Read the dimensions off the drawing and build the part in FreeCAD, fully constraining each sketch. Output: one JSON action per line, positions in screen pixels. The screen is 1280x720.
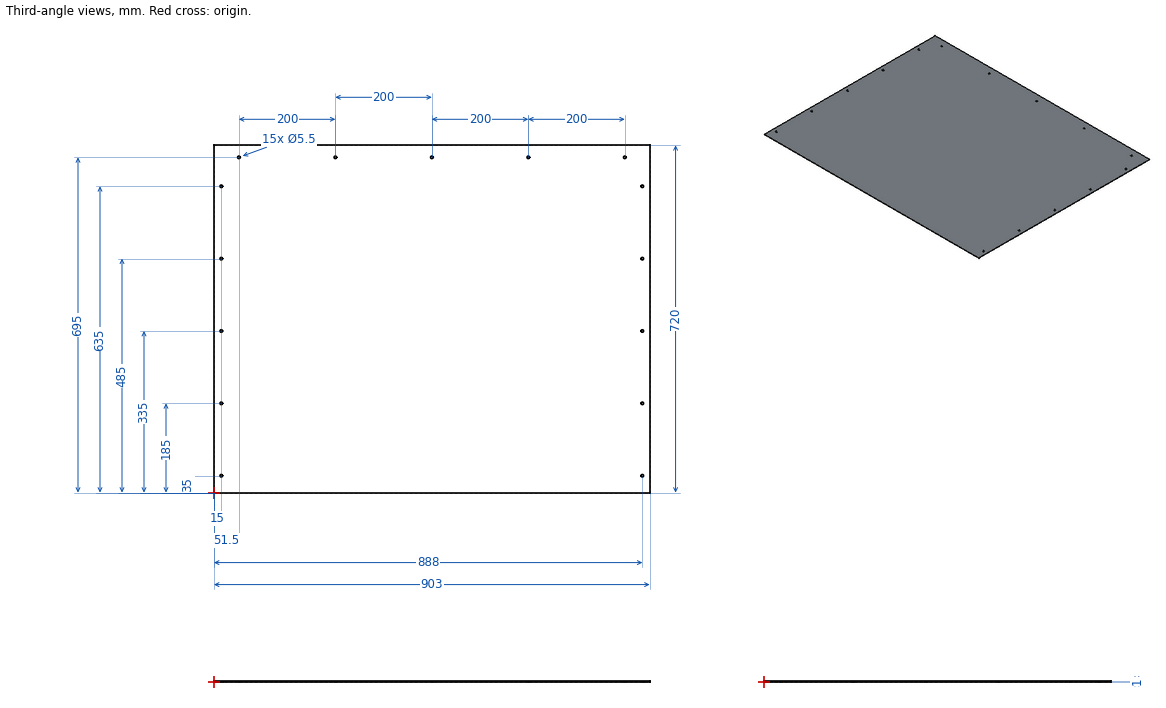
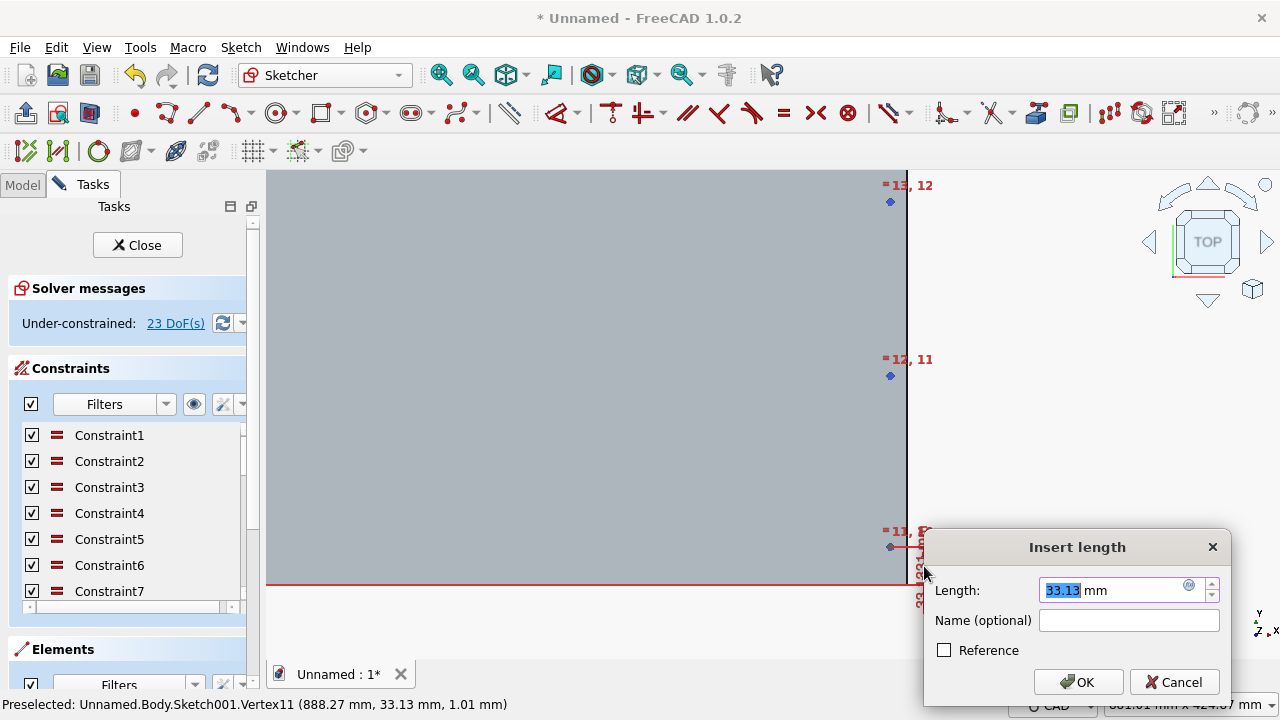
{"action": "type", "text": "35"}
{"action": "key", "text": "Return"}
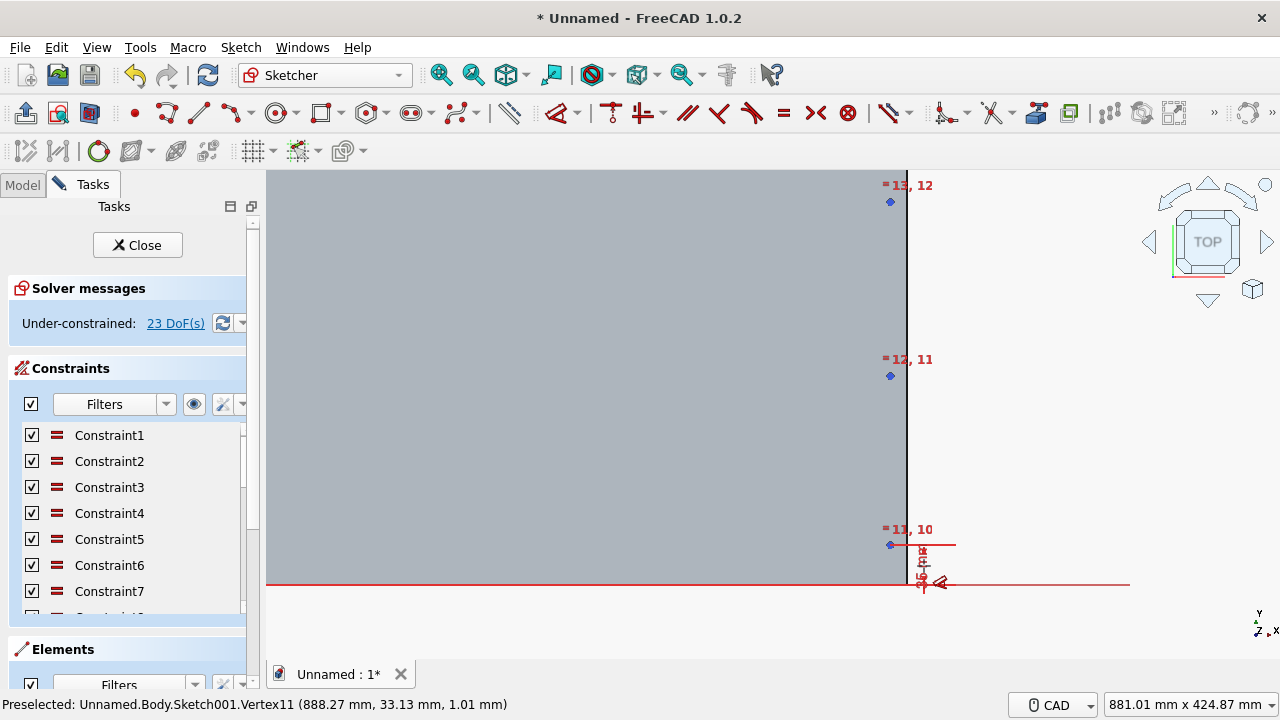
{"action": "scroll", "coordinate": [893, 549], "scroll_direction": "down", "scroll_amount": 5}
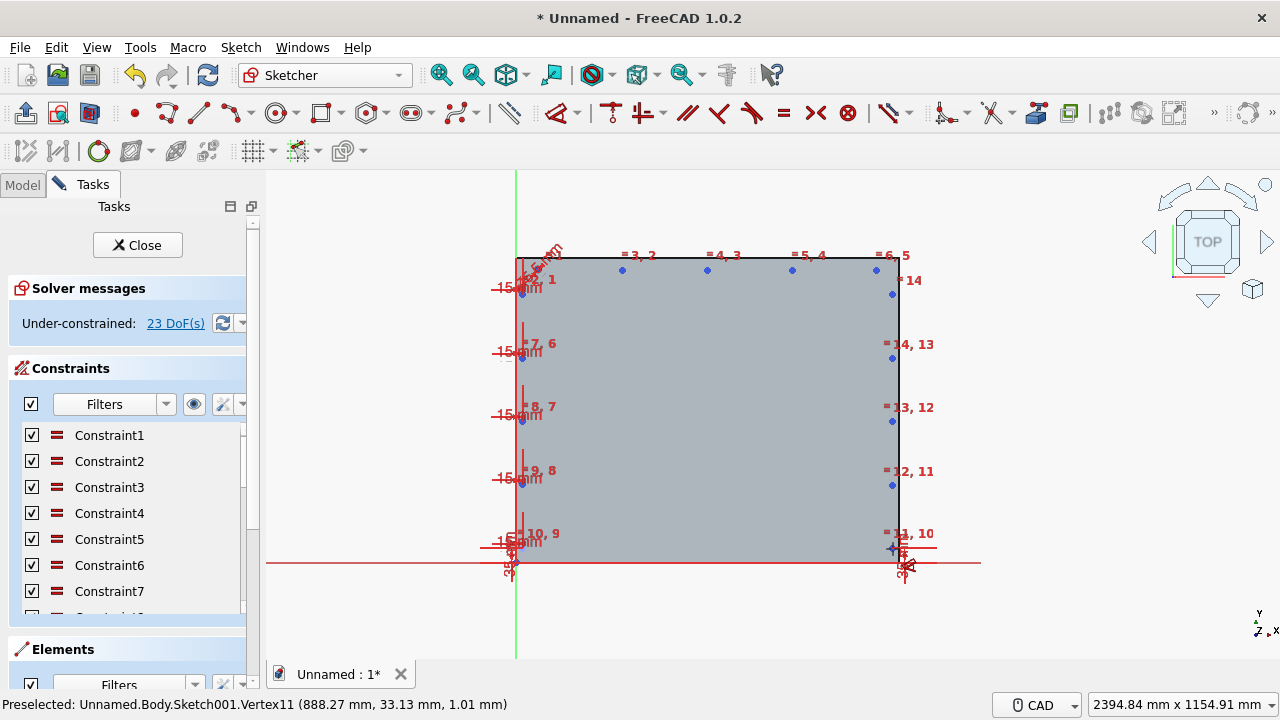
{"action": "left_click", "coordinate": [538, 270]}
{"action": "left_click", "coordinate": [482, 314]}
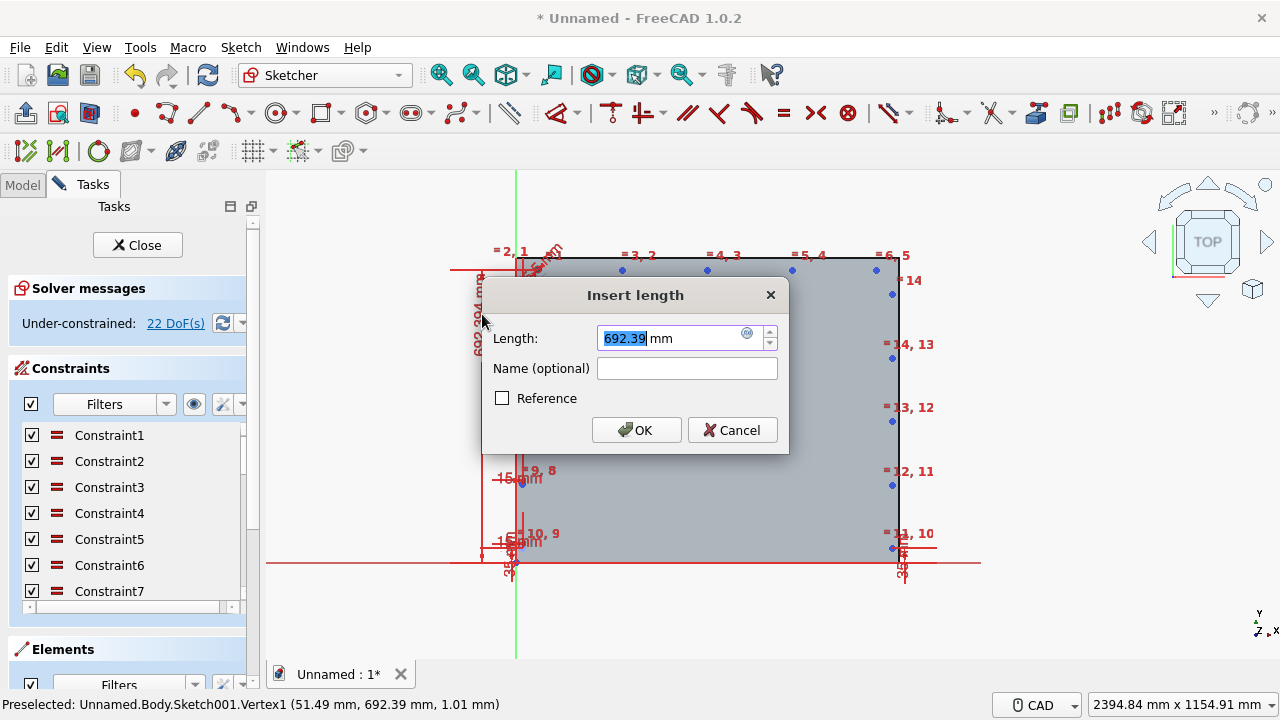
{"action": "type", "text": "695"}
{"action": "key", "text": "Return"}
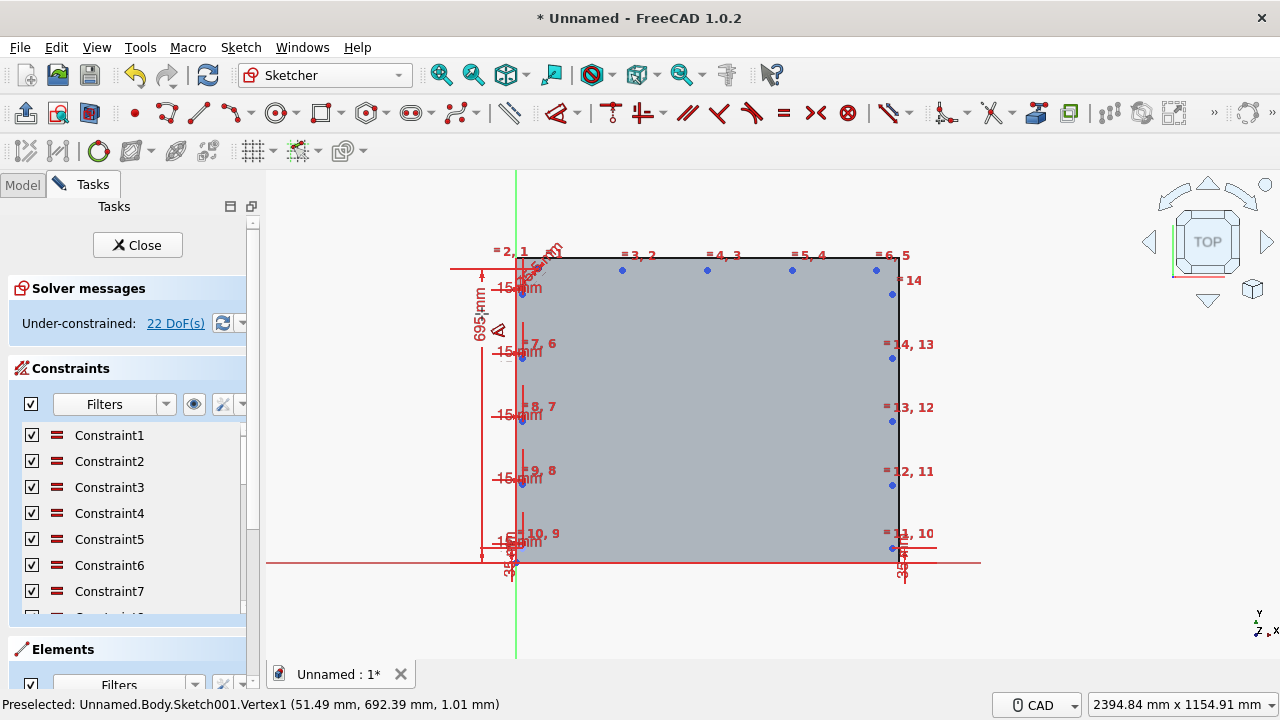
{"action": "left_click", "coordinate": [523, 294]}
{"action": "left_click", "coordinate": [482, 523]}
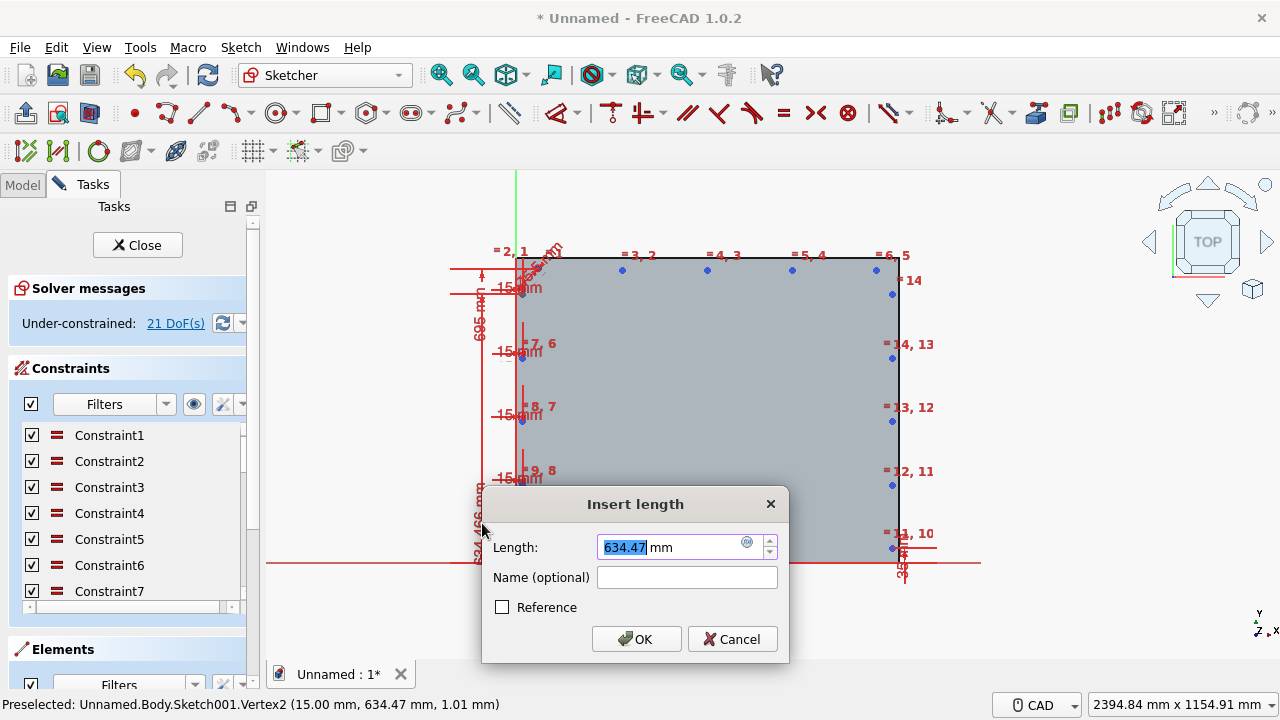
{"action": "type", "text": "635"}
{"action": "key", "text": "Return"}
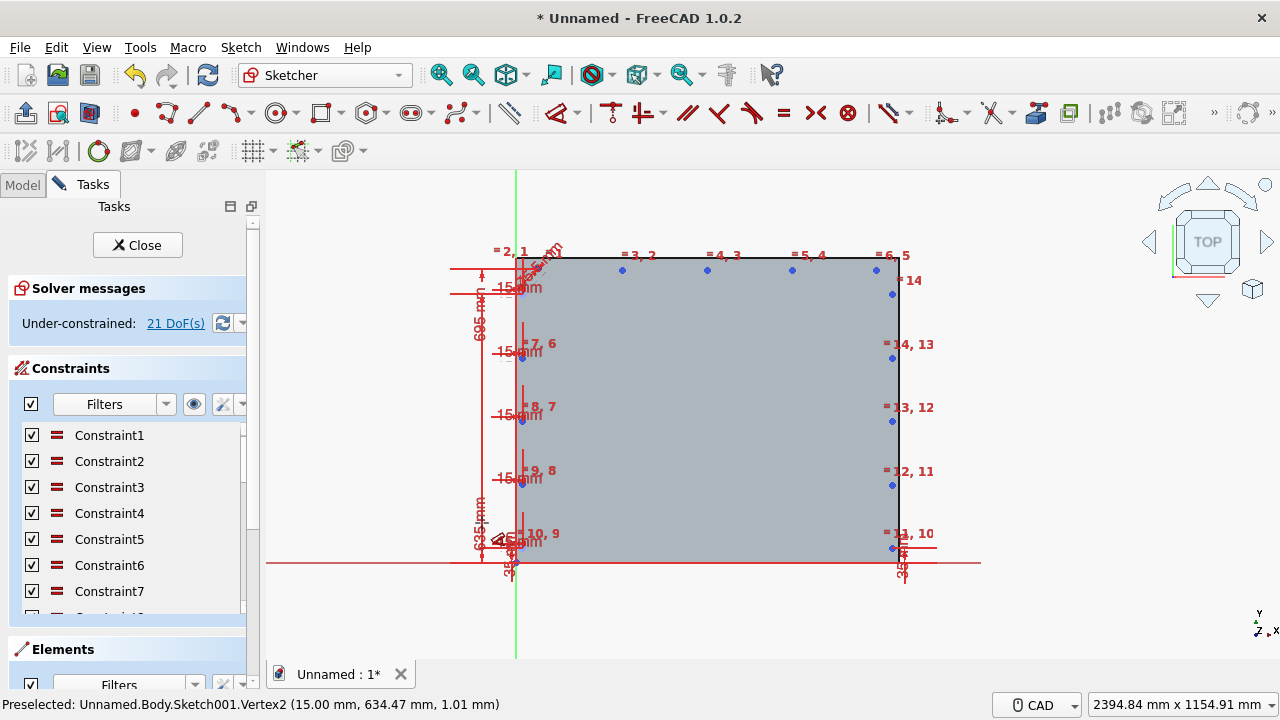
{"action": "left_click", "coordinate": [622, 270]}
{"action": "left_click", "coordinate": [656, 416]}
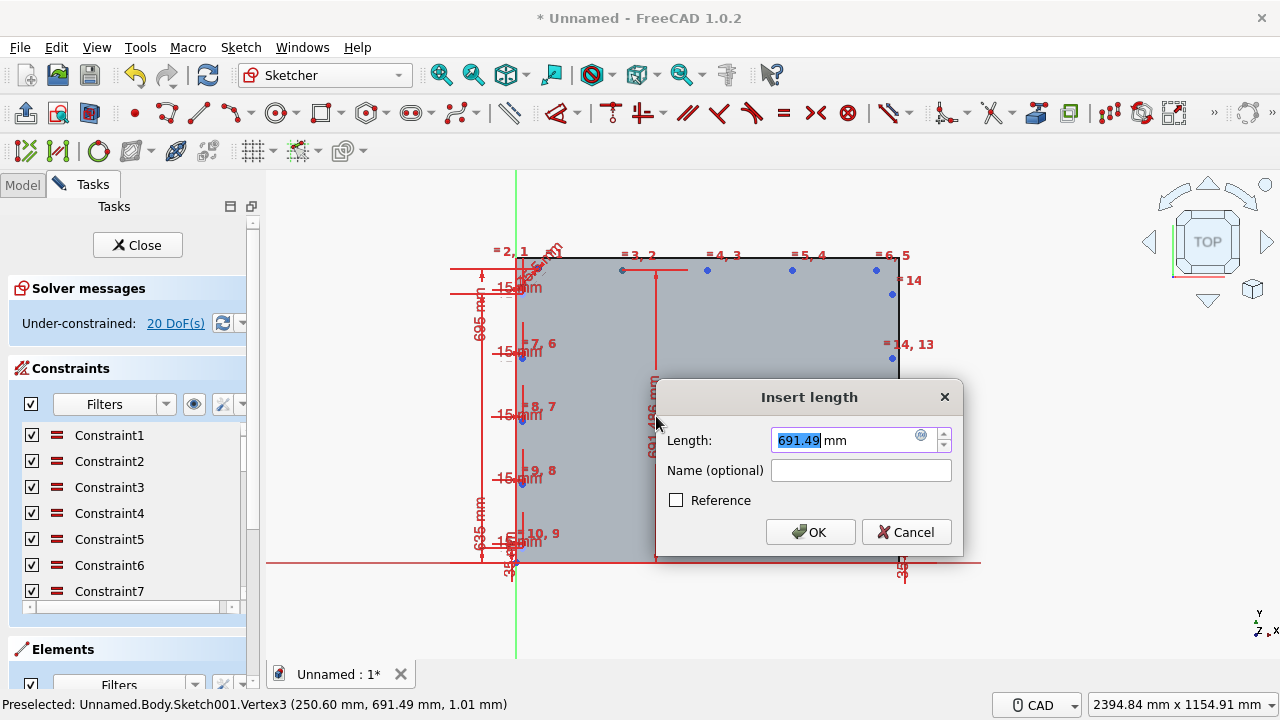
{"action": "type", "text": "695"}
{"action": "key", "text": "Return"}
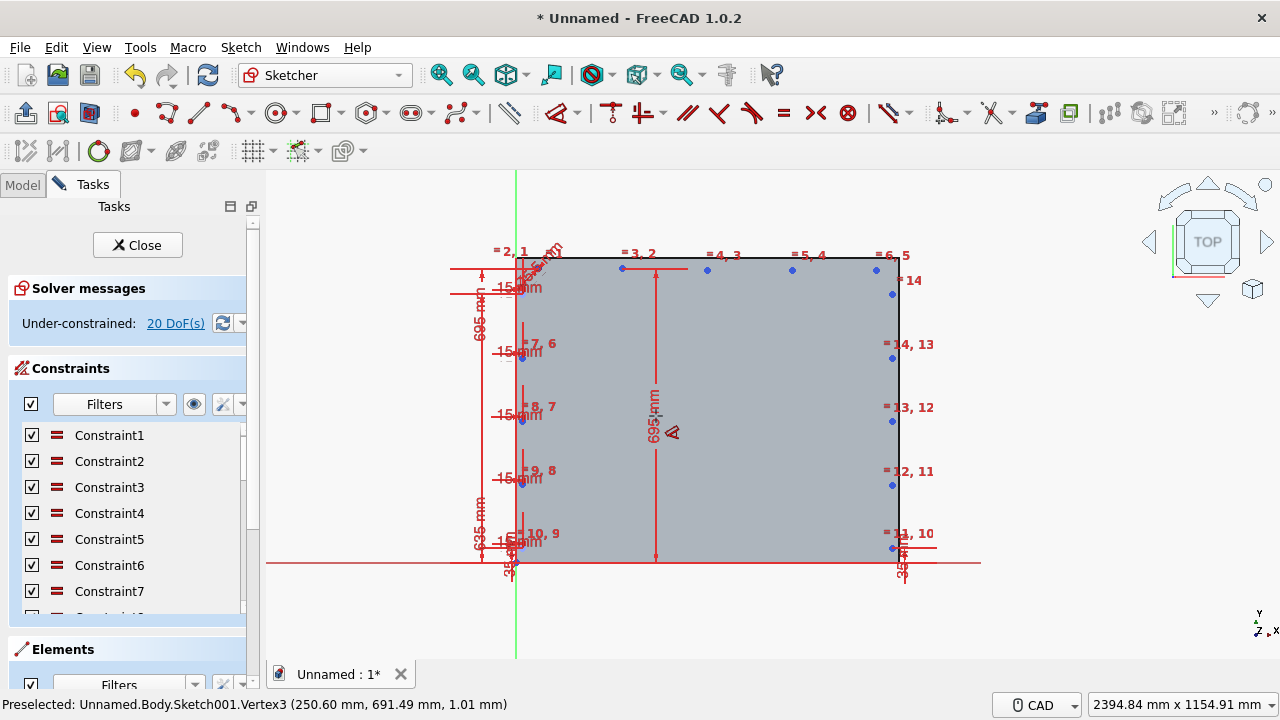
{"action": "left_click", "coordinate": [707, 270]}
{"action": "left_click", "coordinate": [741, 416]}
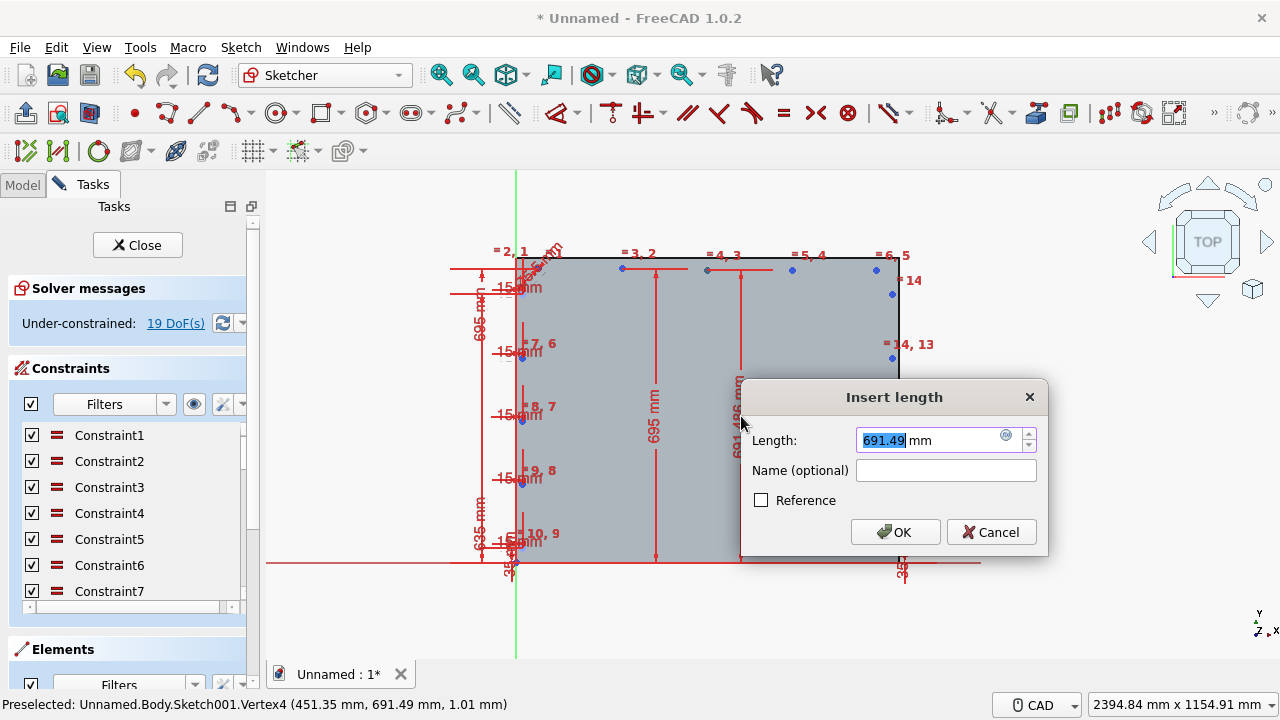
{"action": "type", "text": "695"}
{"action": "key", "text": "Return"}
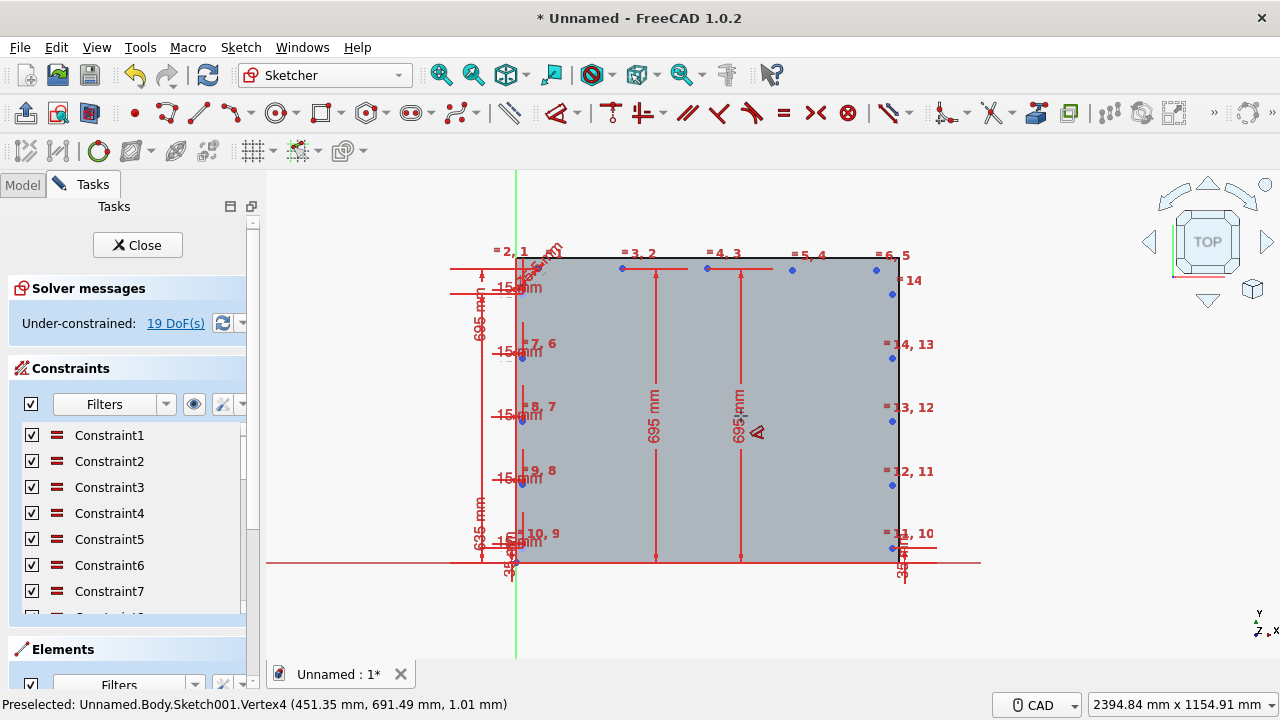
{"action": "left_click", "coordinate": [793, 270]}
{"action": "left_click", "coordinate": [827, 416]}